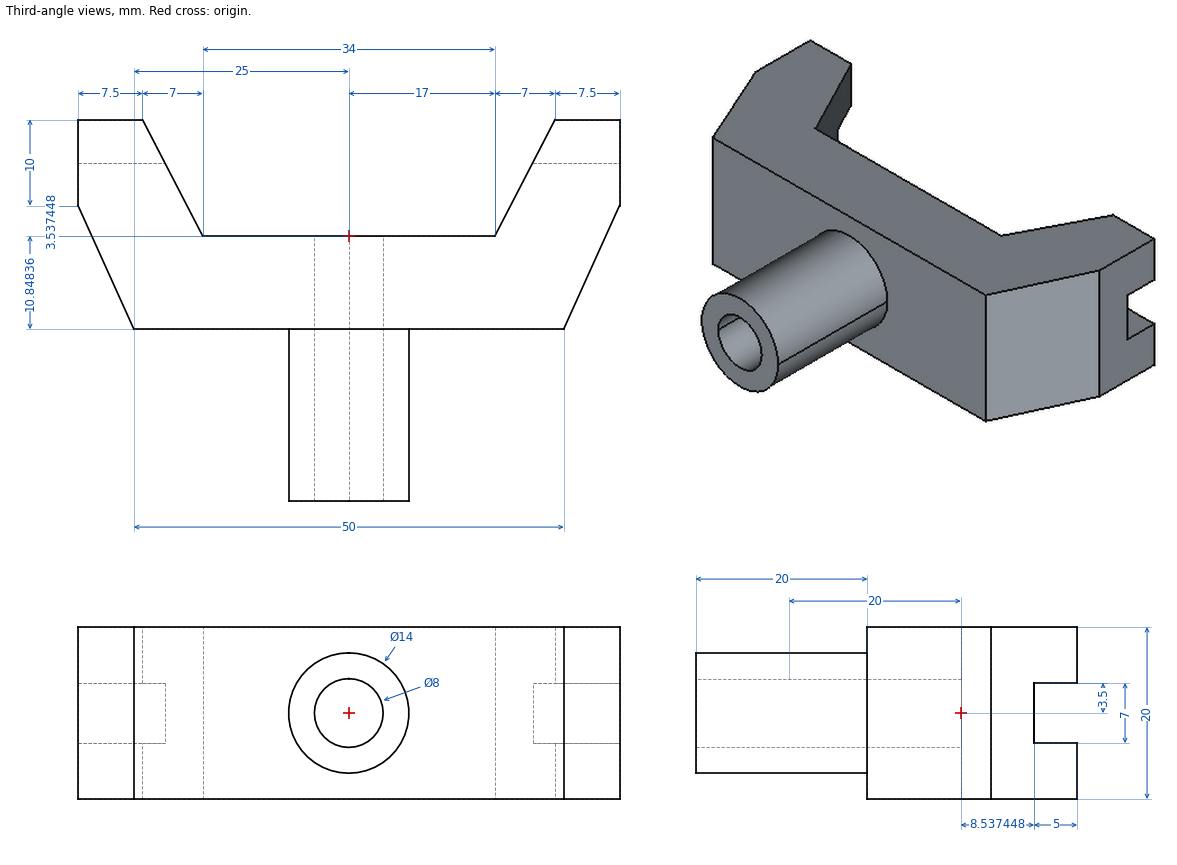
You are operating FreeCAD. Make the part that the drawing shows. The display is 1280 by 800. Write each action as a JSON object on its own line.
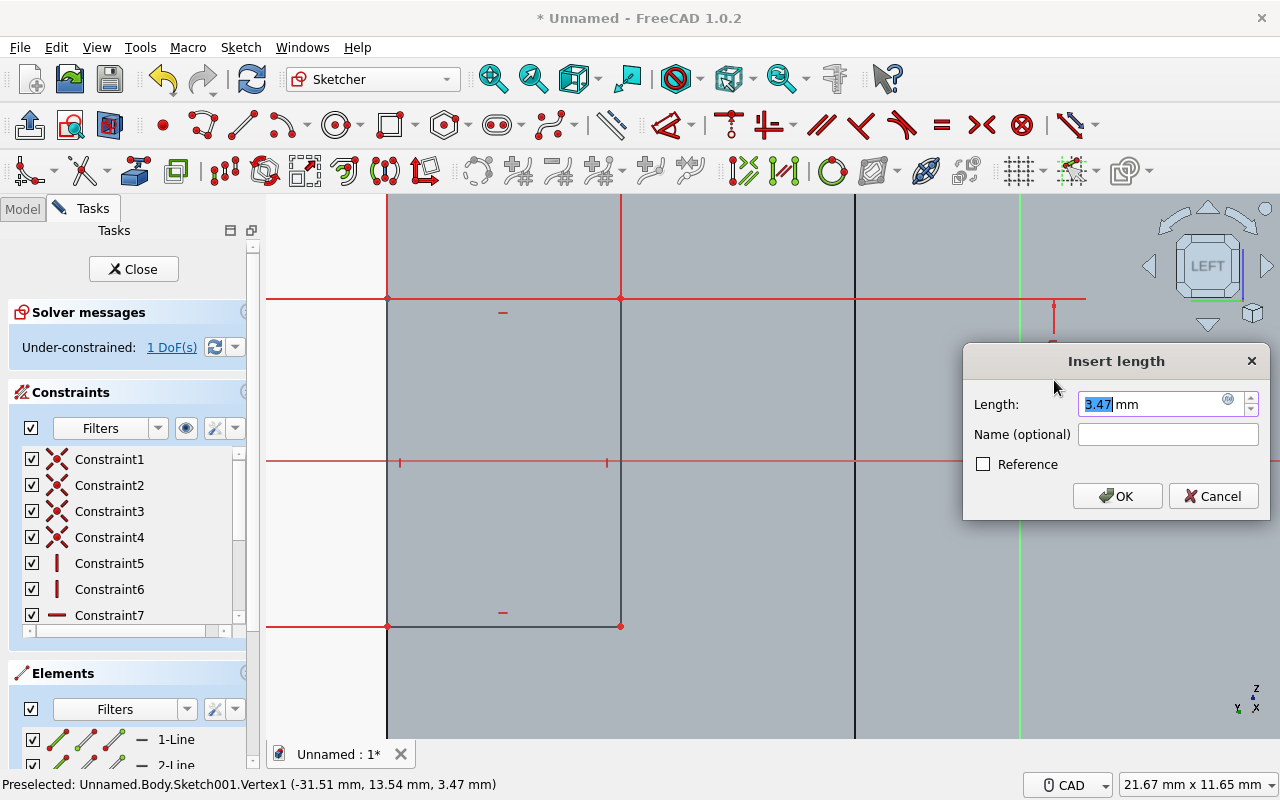
{"action": "type", "text": "3.5"}
{"action": "key", "text": "Return"}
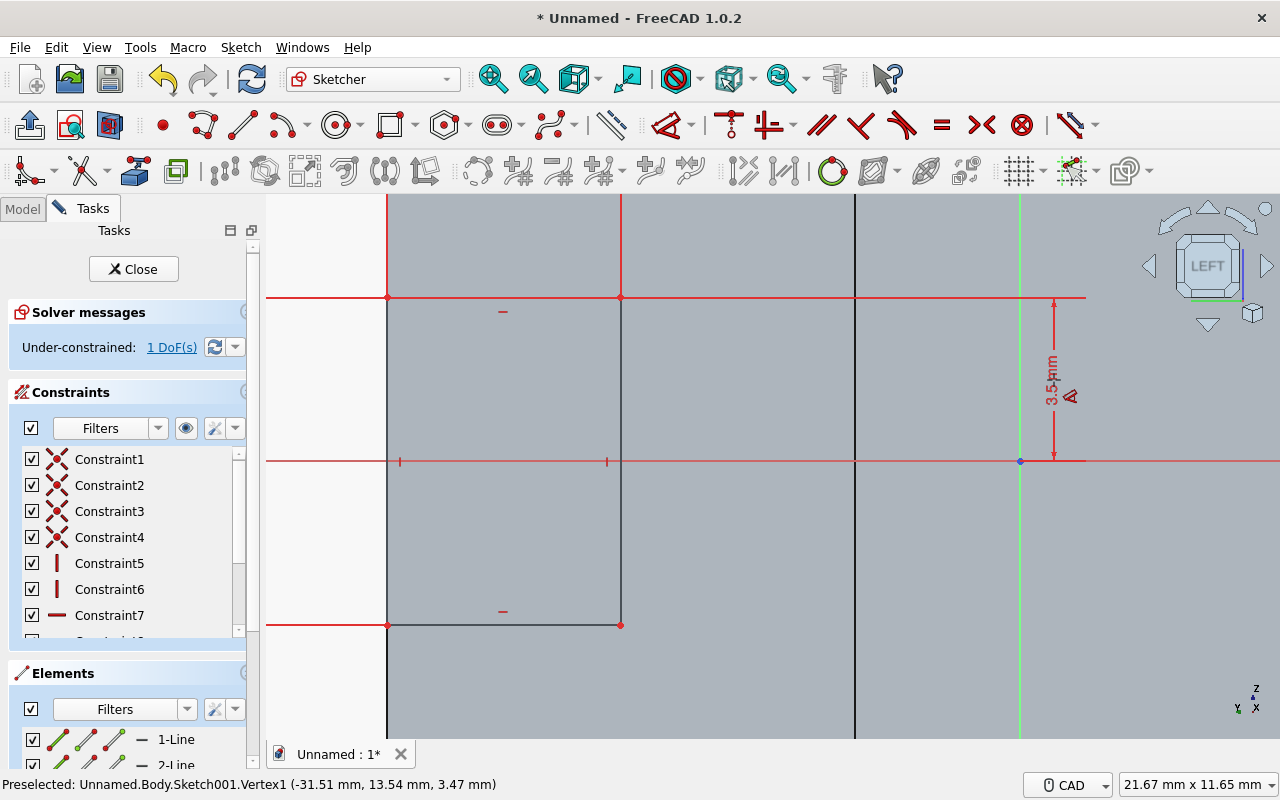
{"action": "left_click", "coordinate": [621, 625]}
{"action": "left_click", "coordinate": [821, 659]}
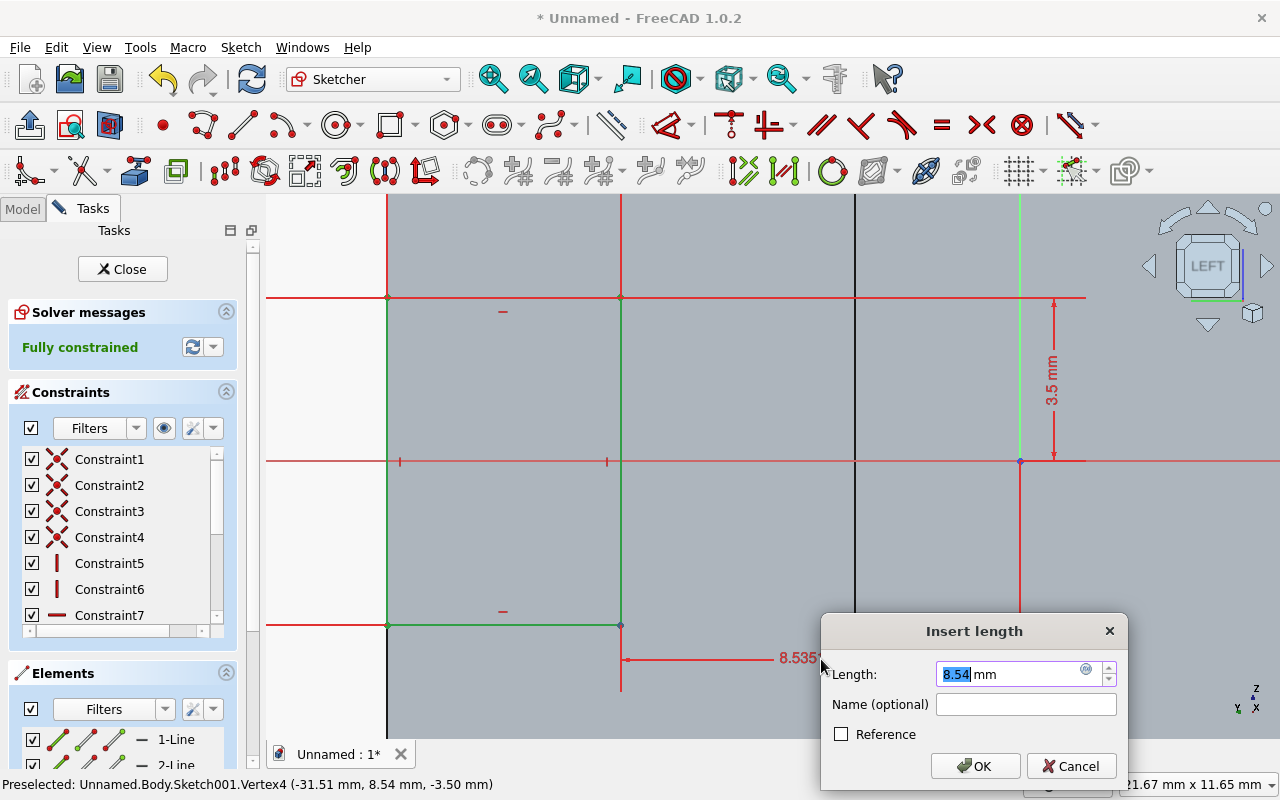
{"action": "type", "text": "8.537448"}
{"action": "key", "text": "Return"}
{"action": "key", "text": "Escape"}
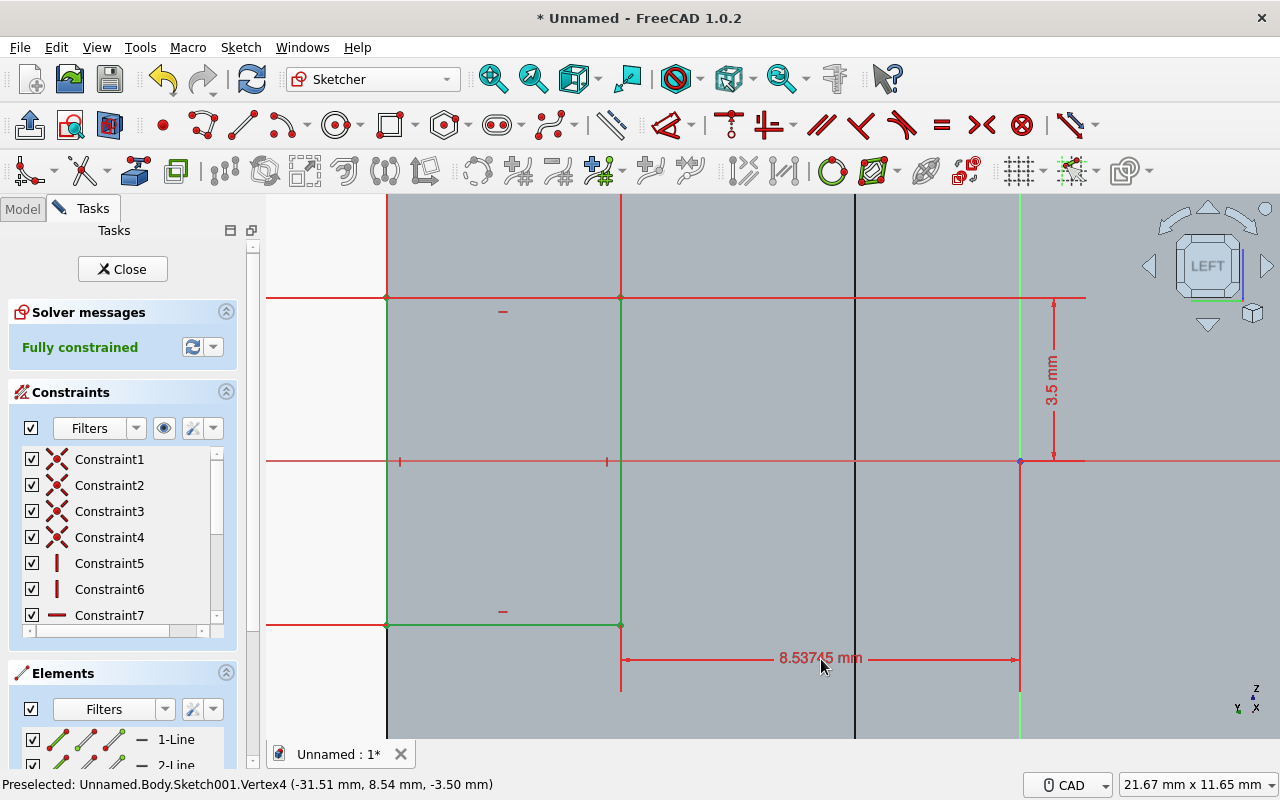
{"action": "left_click", "coordinate": [123, 269]}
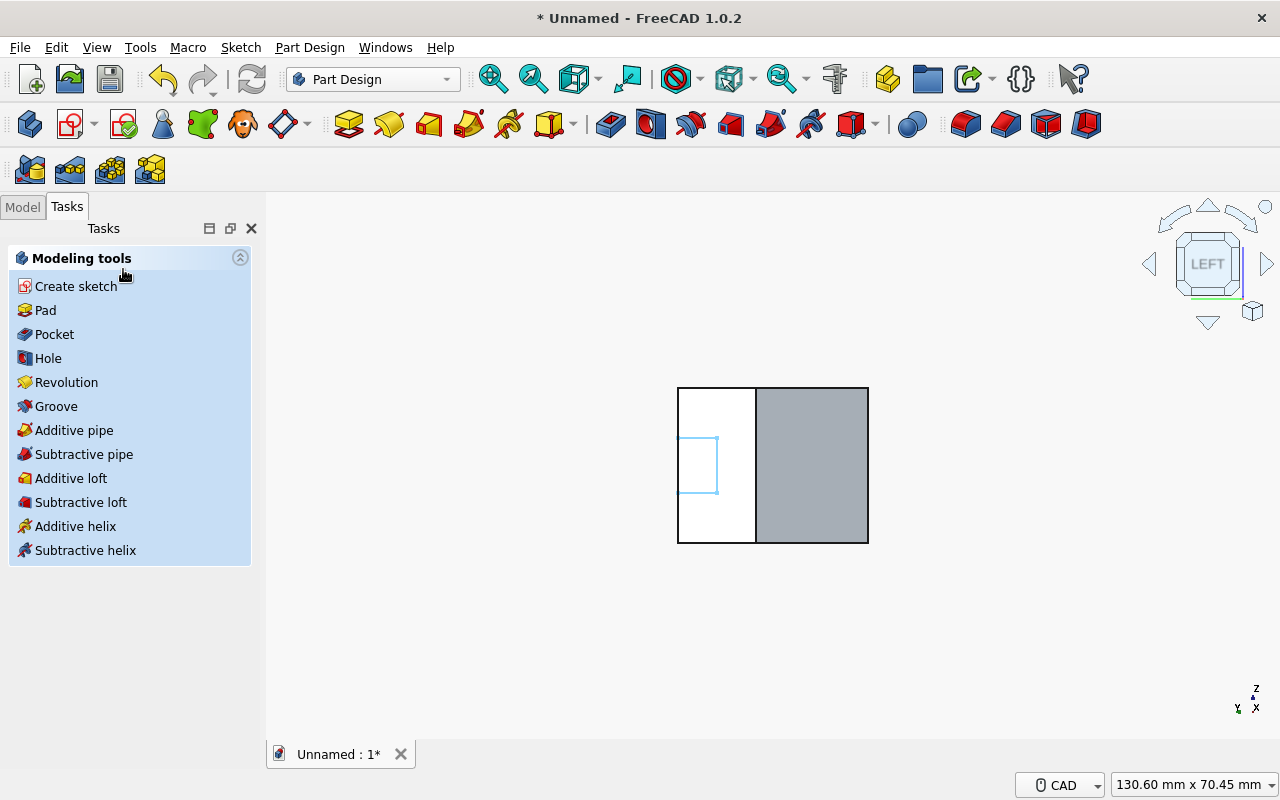
{"action": "left_click", "coordinate": [612, 124]}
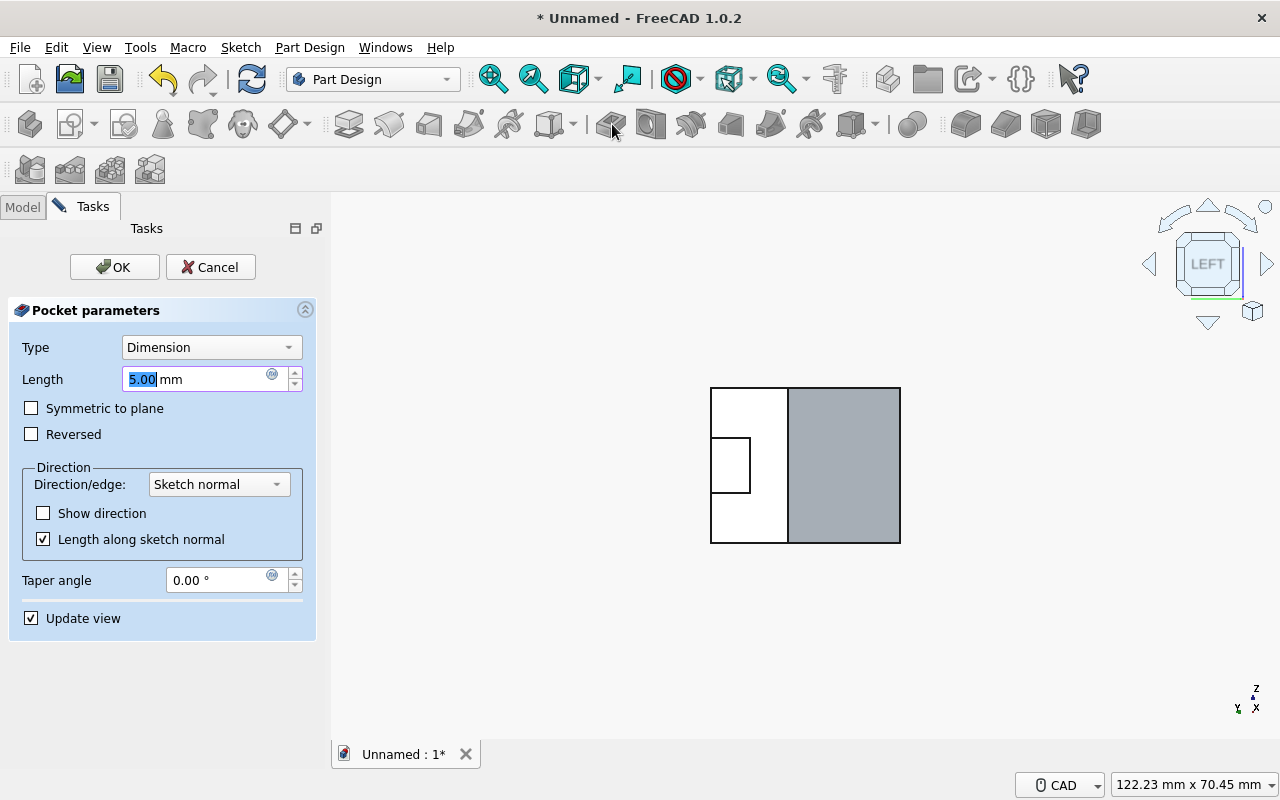
{"action": "left_click", "coordinate": [212, 348]}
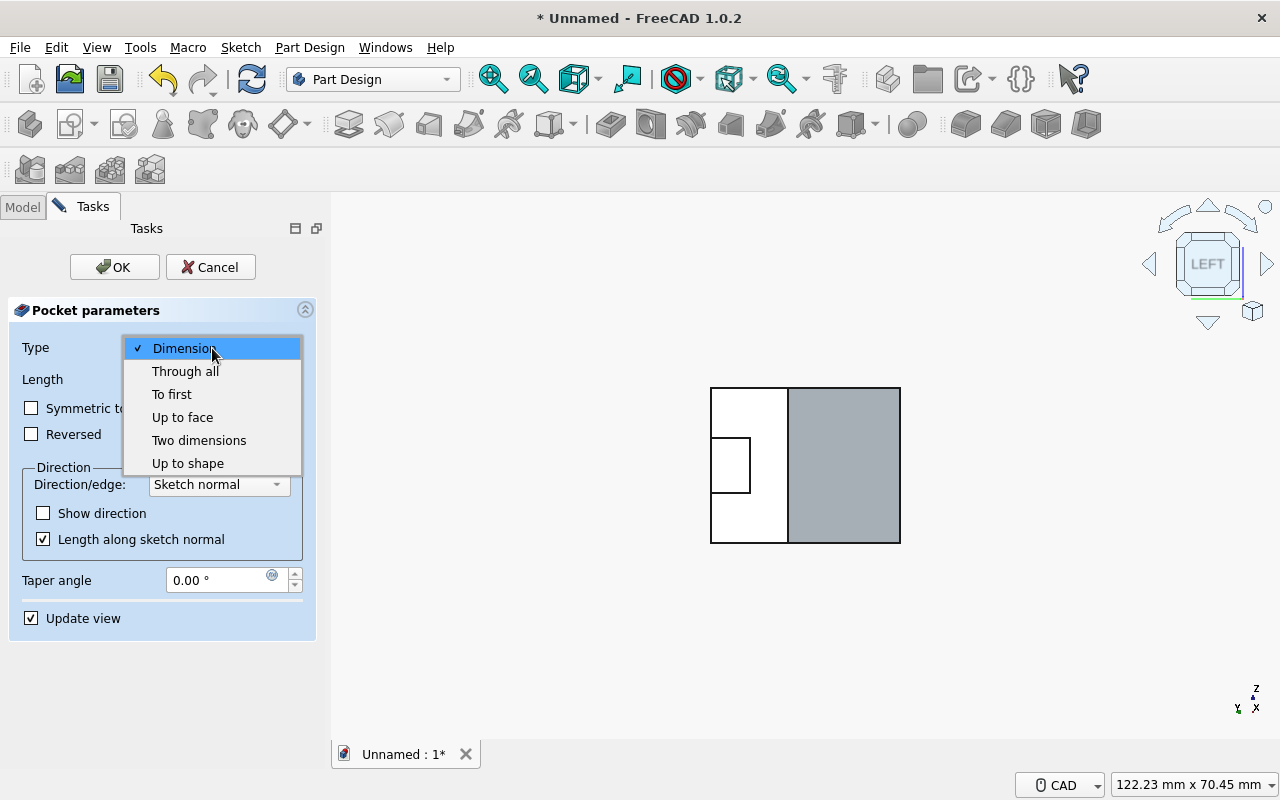
{"action": "left_click", "coordinate": [212, 372]}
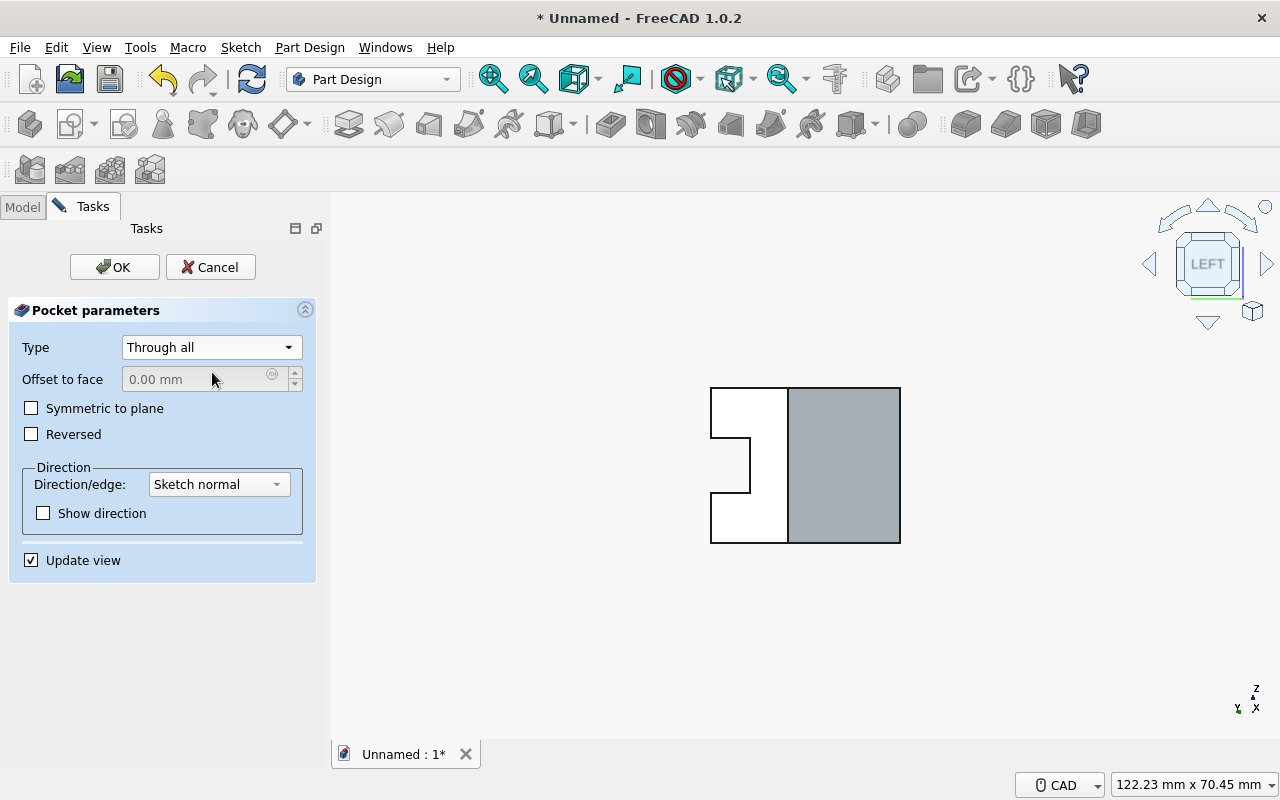
{"action": "left_click", "coordinate": [115, 267]}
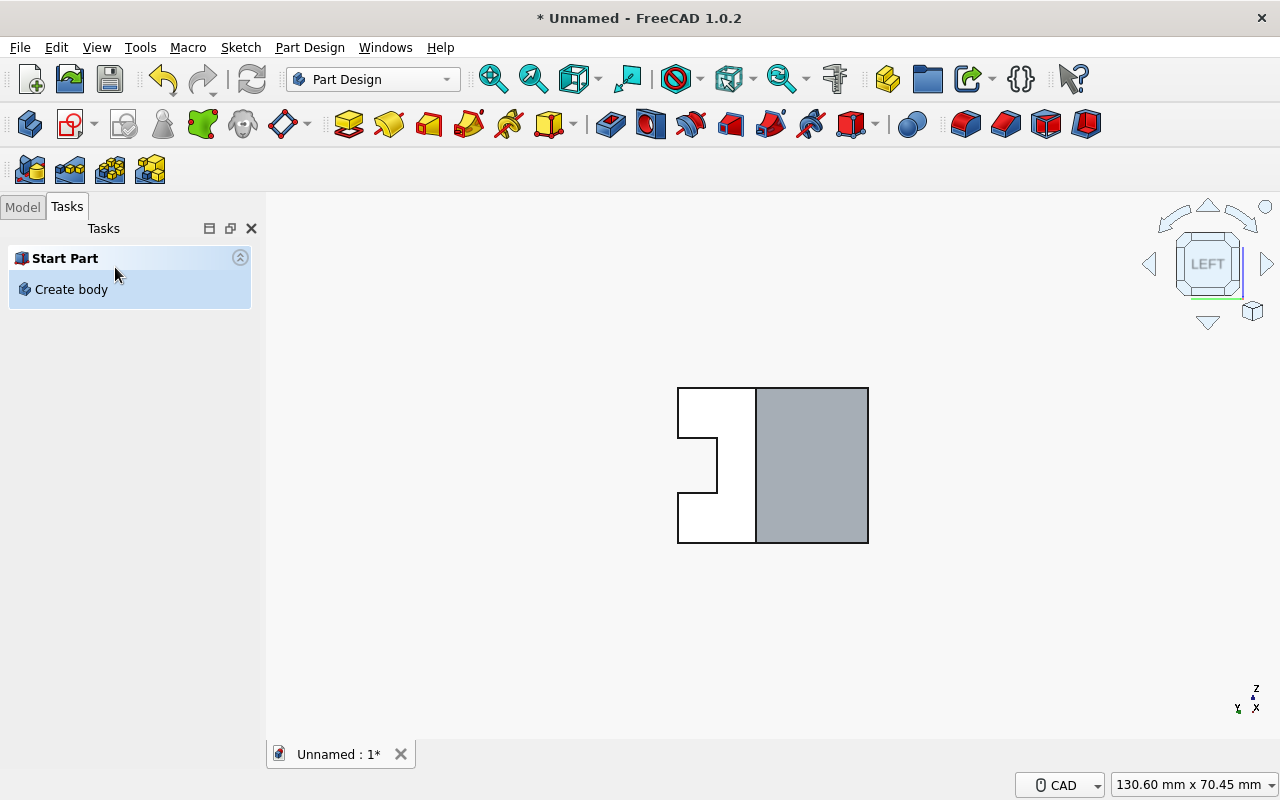
{"action": "left_click", "coordinate": [494, 80]}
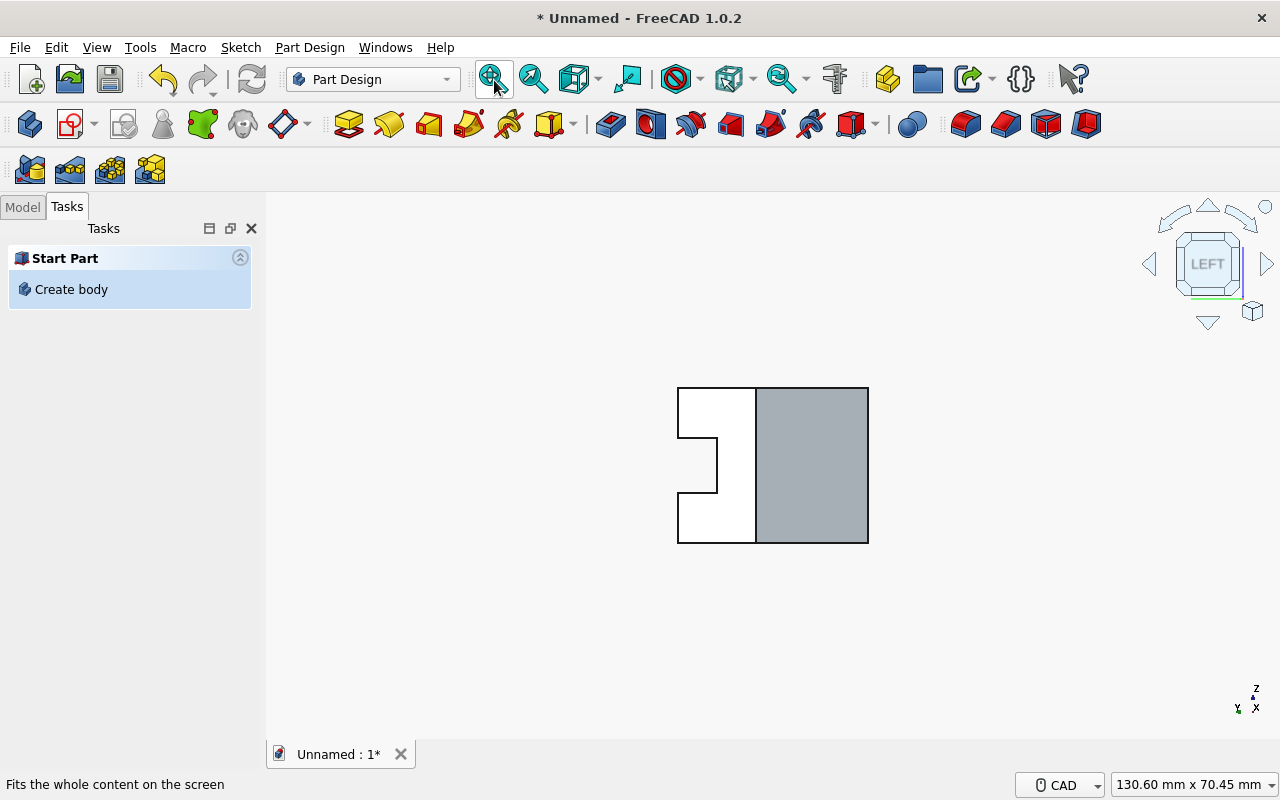
{"action": "left_click", "coordinate": [70, 124]}